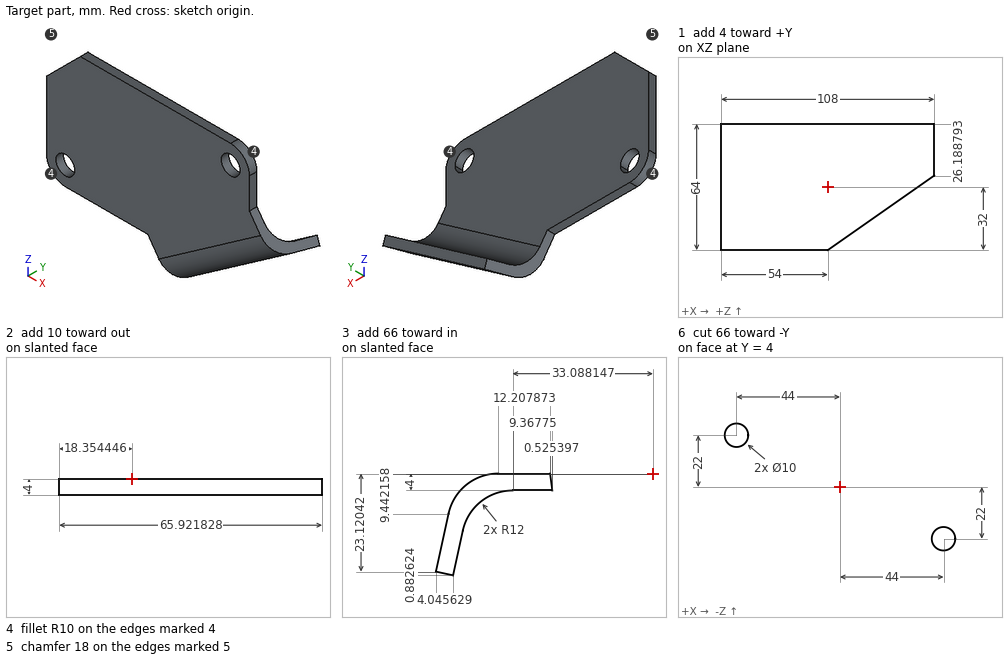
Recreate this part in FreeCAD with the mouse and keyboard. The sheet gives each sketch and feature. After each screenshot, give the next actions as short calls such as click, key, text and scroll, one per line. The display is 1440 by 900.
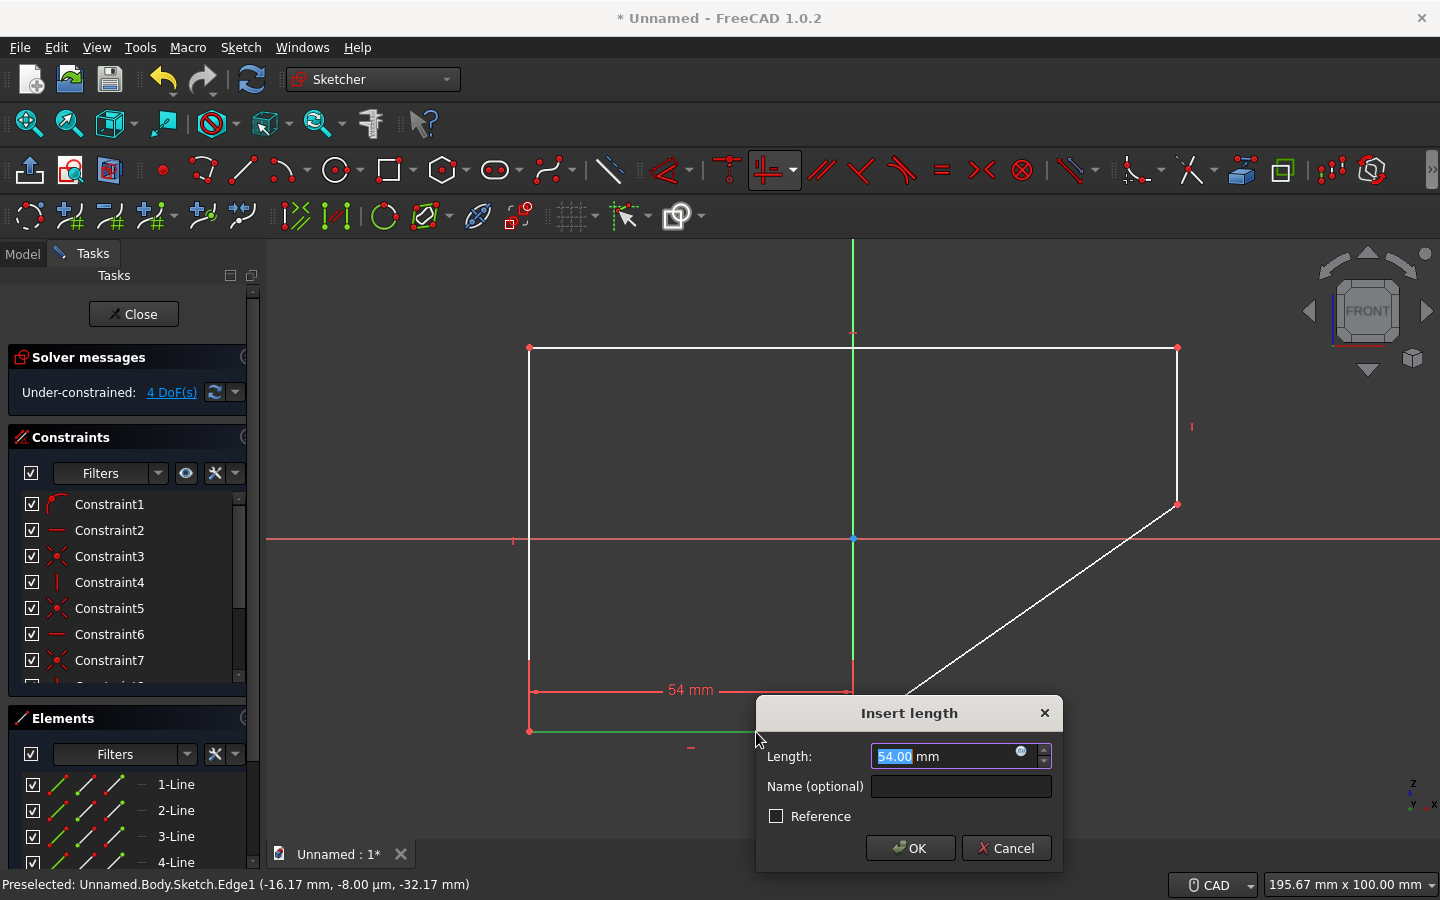
text(54)
key(Return)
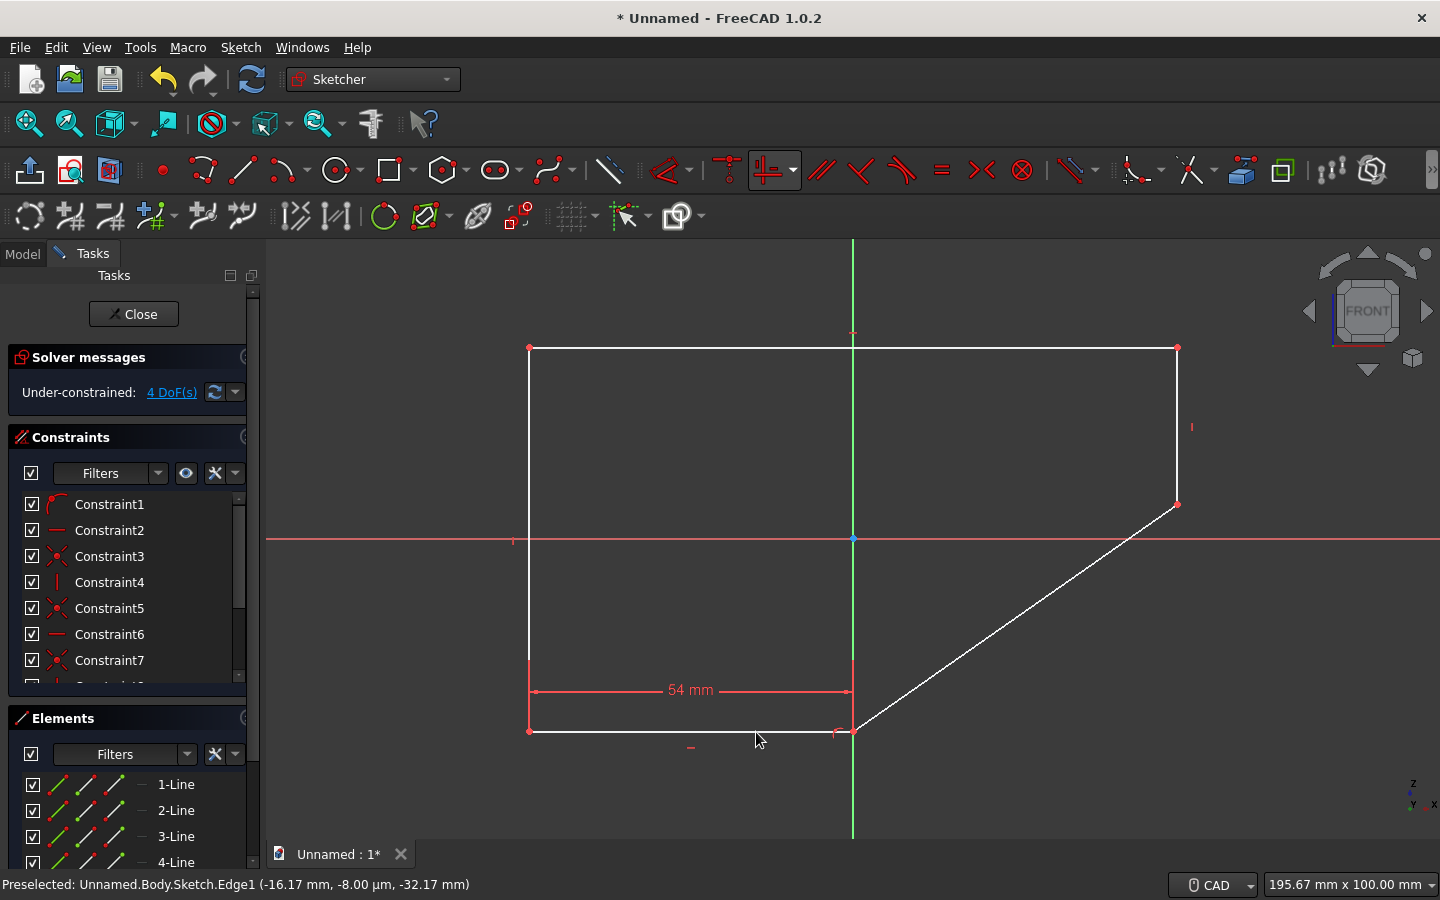
click(529, 617)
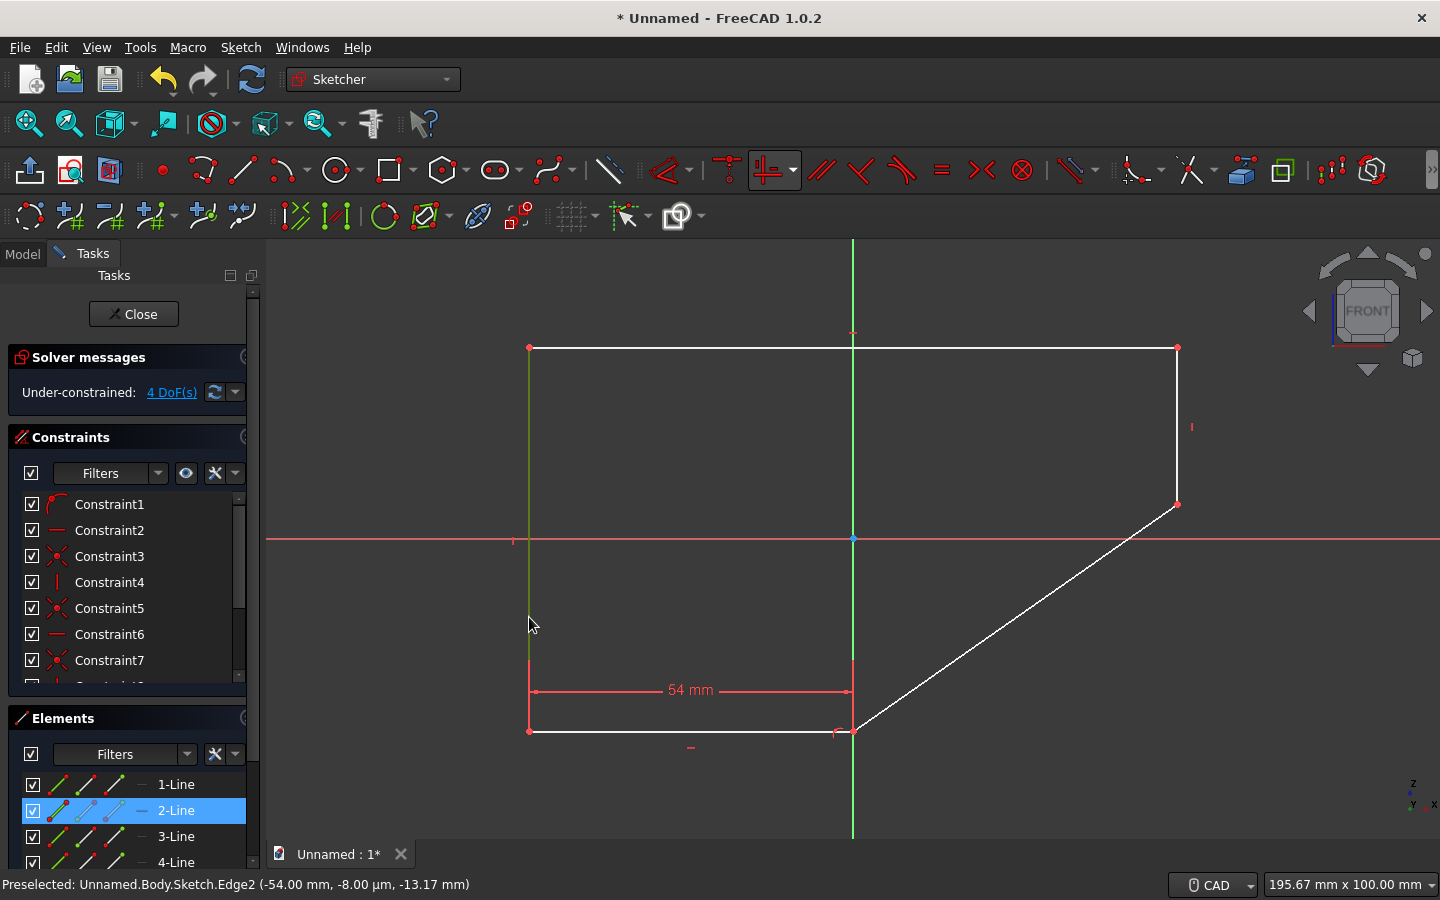
key(i)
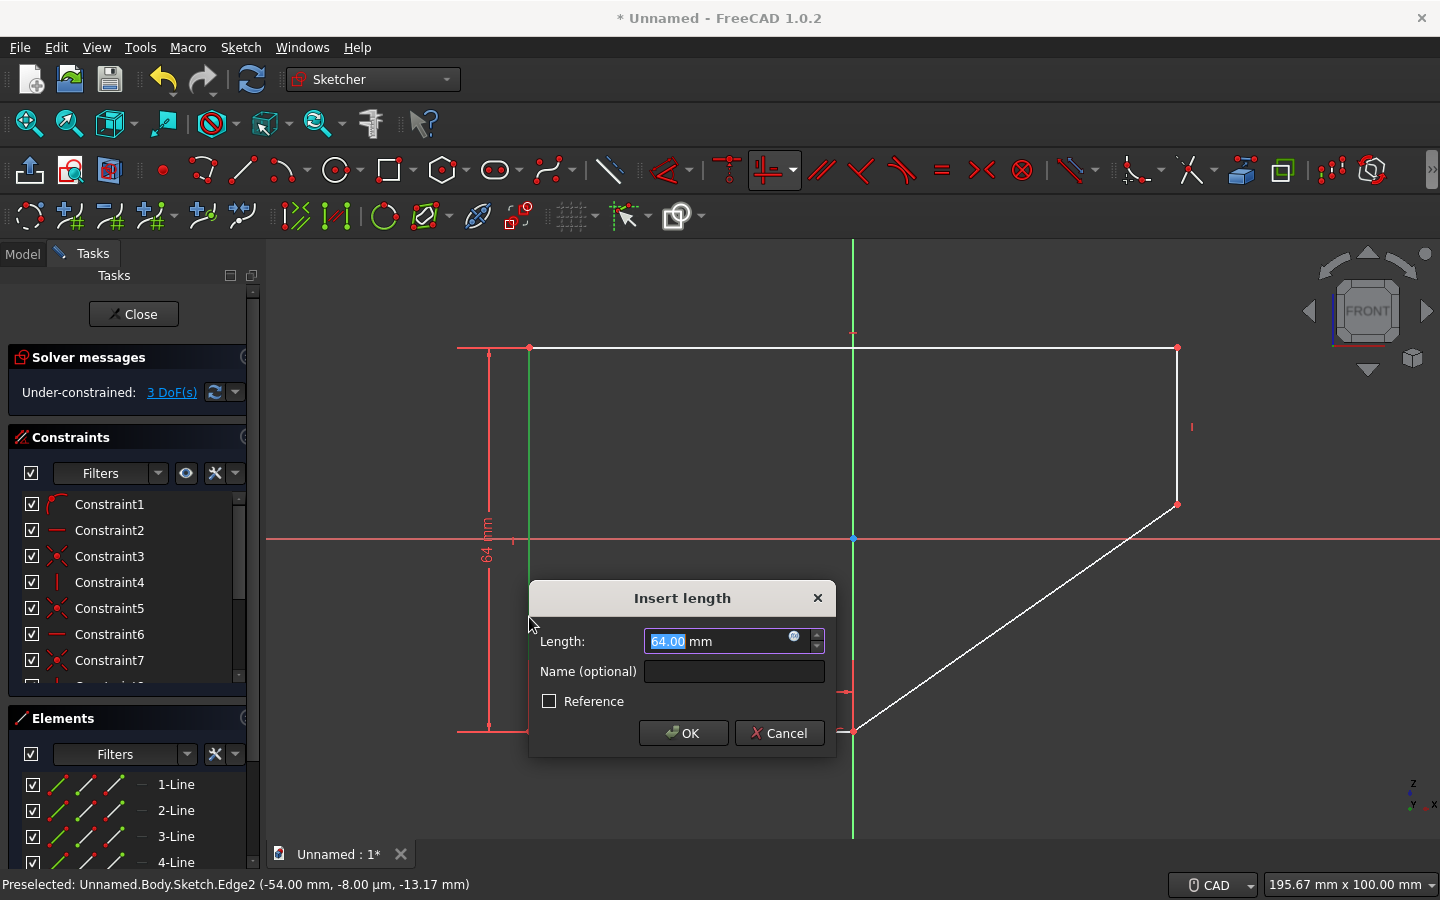
text(64)
key(Return)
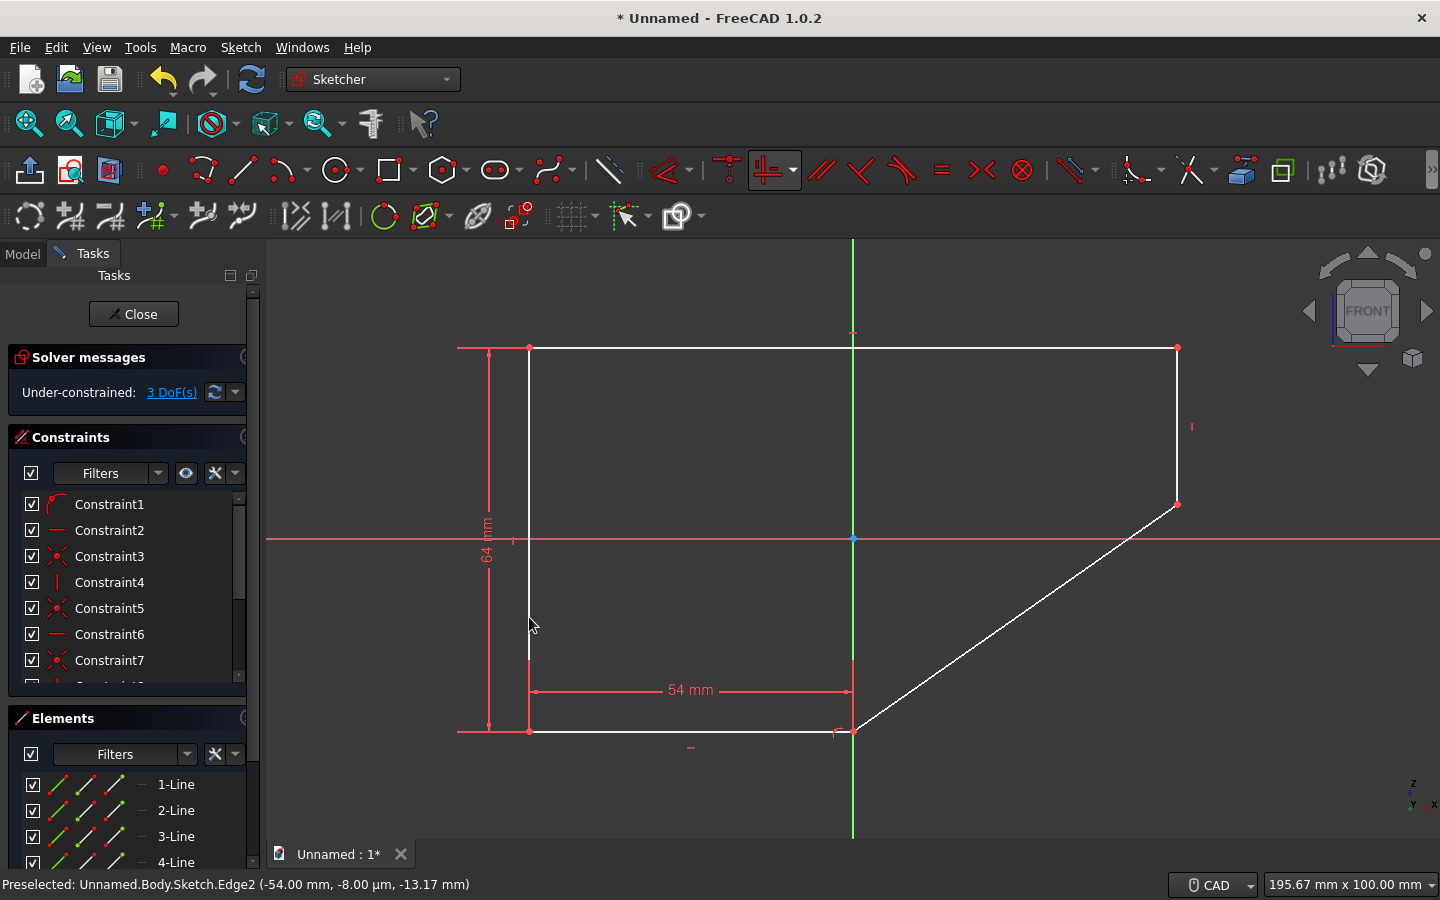
click(723, 348)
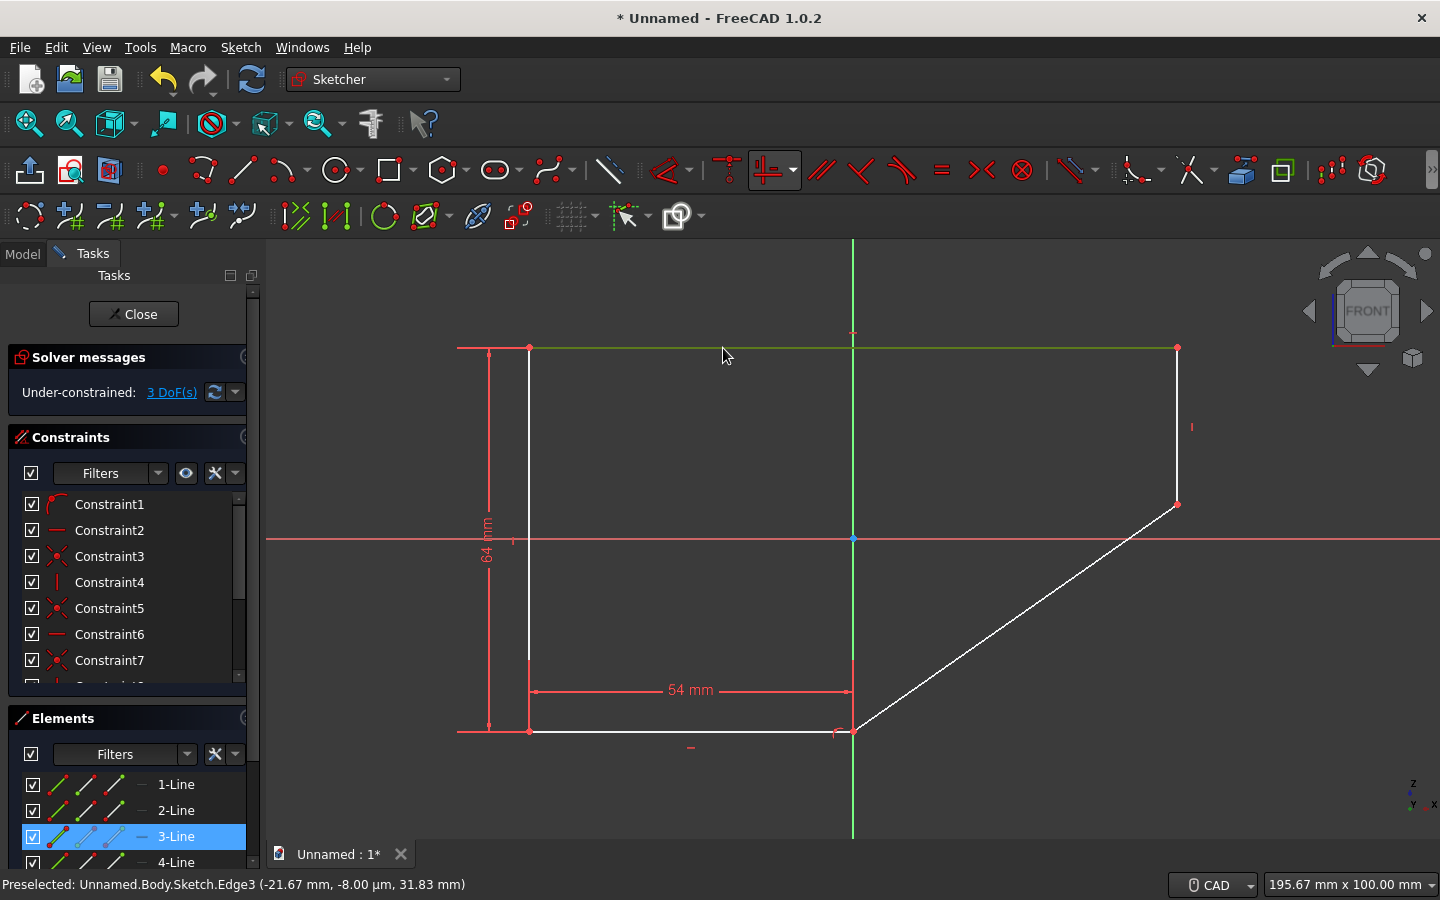
key(l)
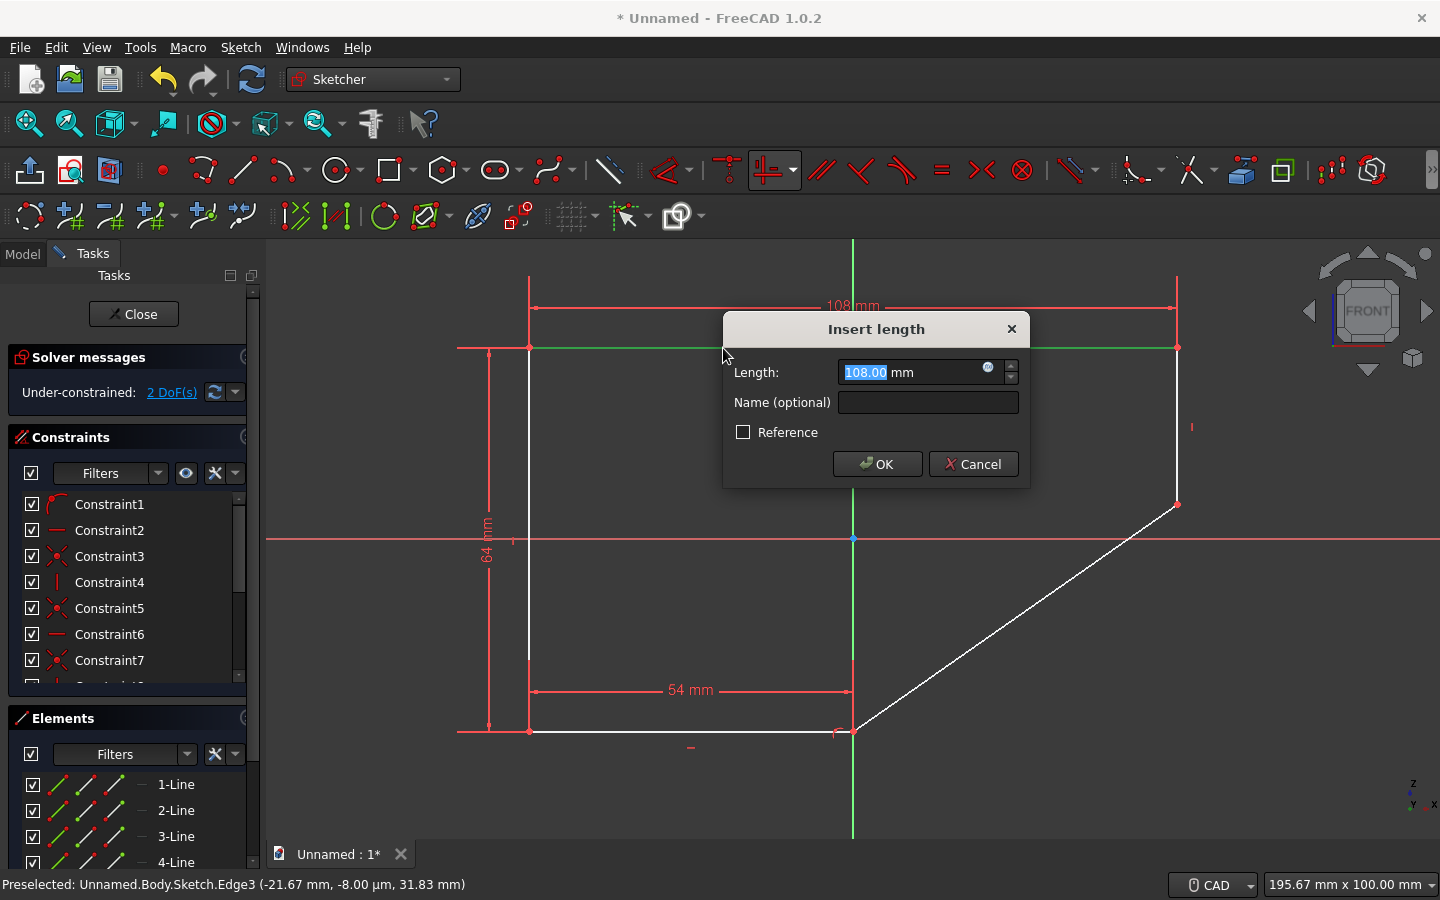
text(108)
key(Return)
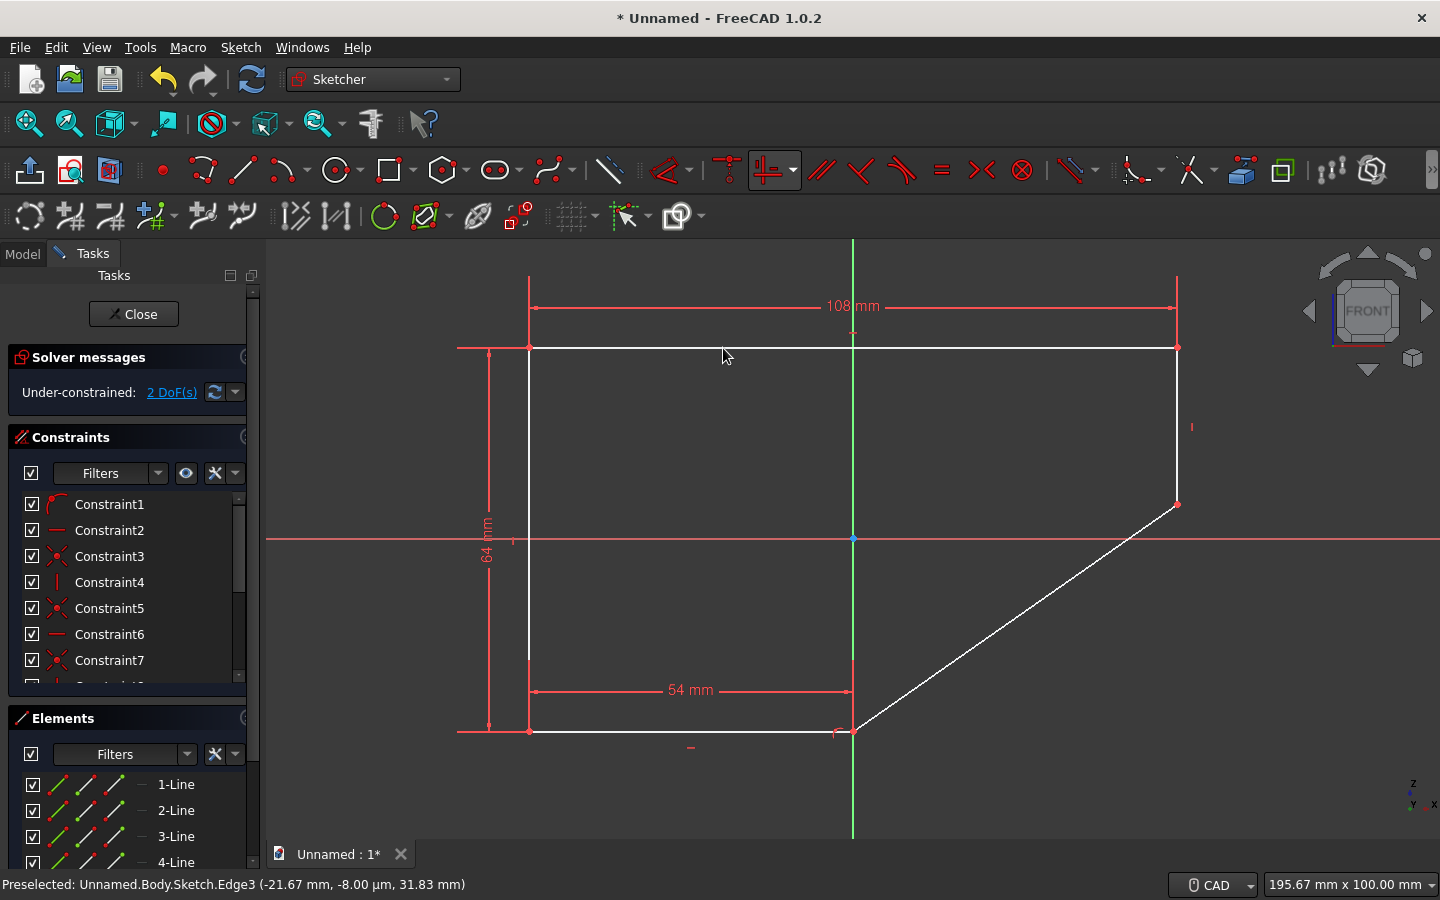
click(853, 732)